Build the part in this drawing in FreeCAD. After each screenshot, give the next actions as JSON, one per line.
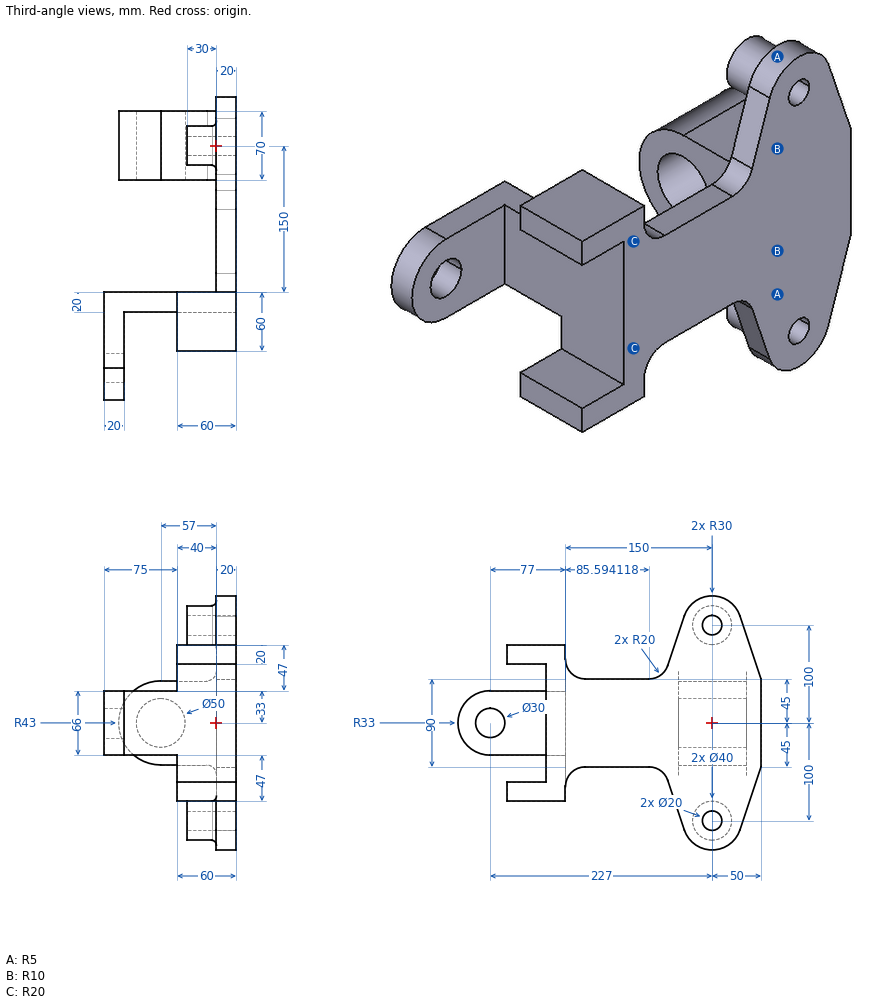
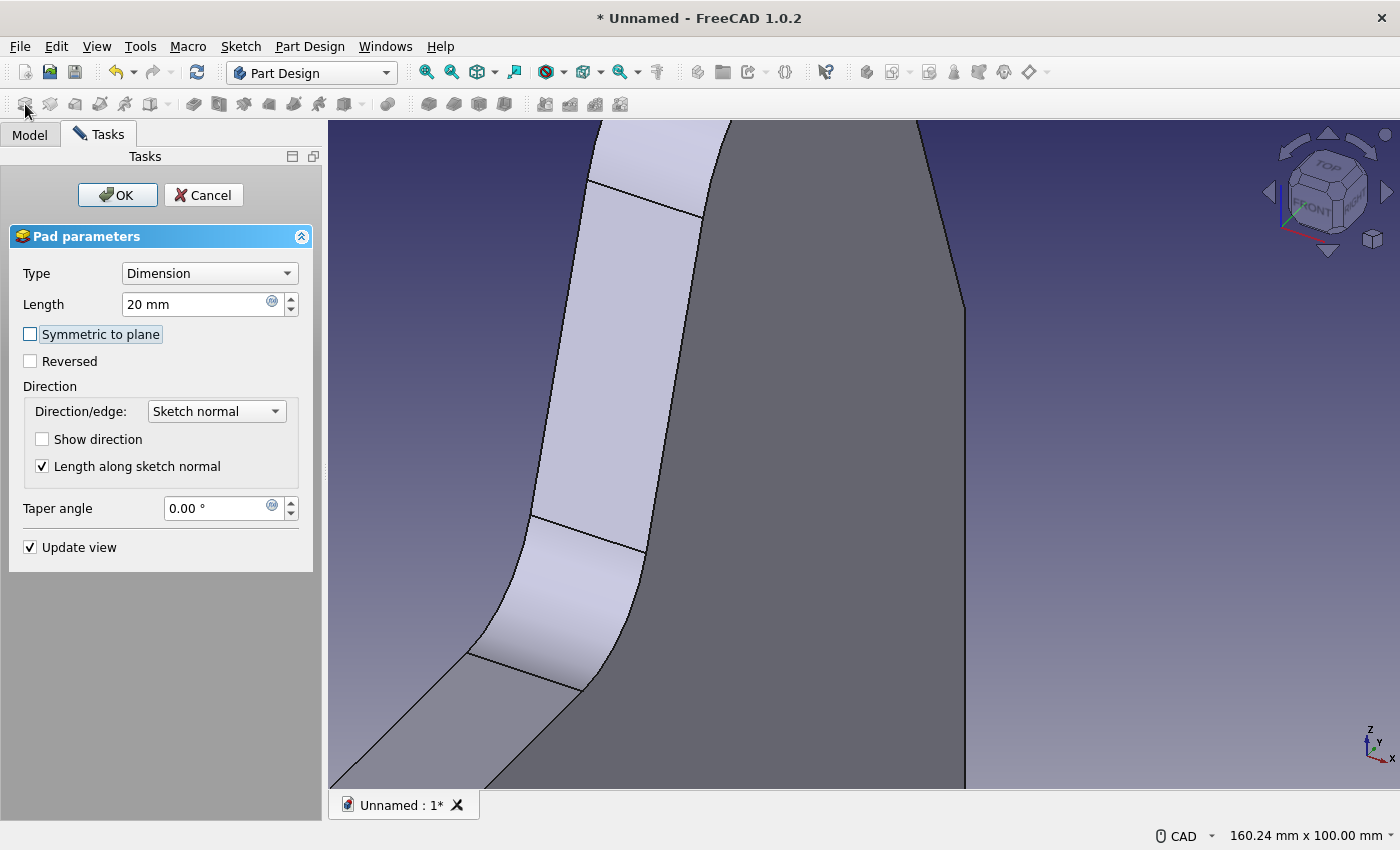
{"action": "left_click", "coordinate": [118, 195]}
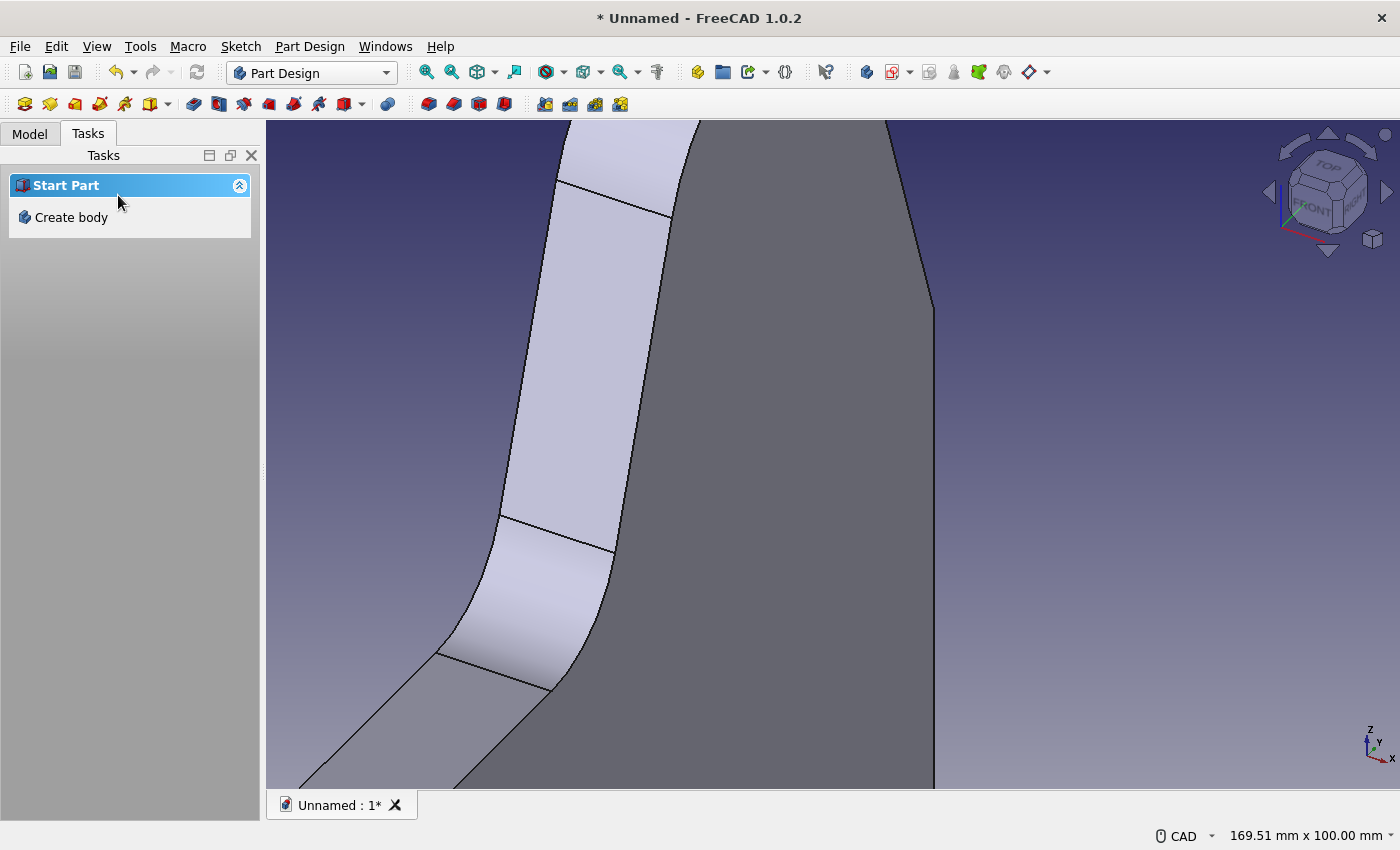
{"action": "left_click", "coordinate": [427, 72]}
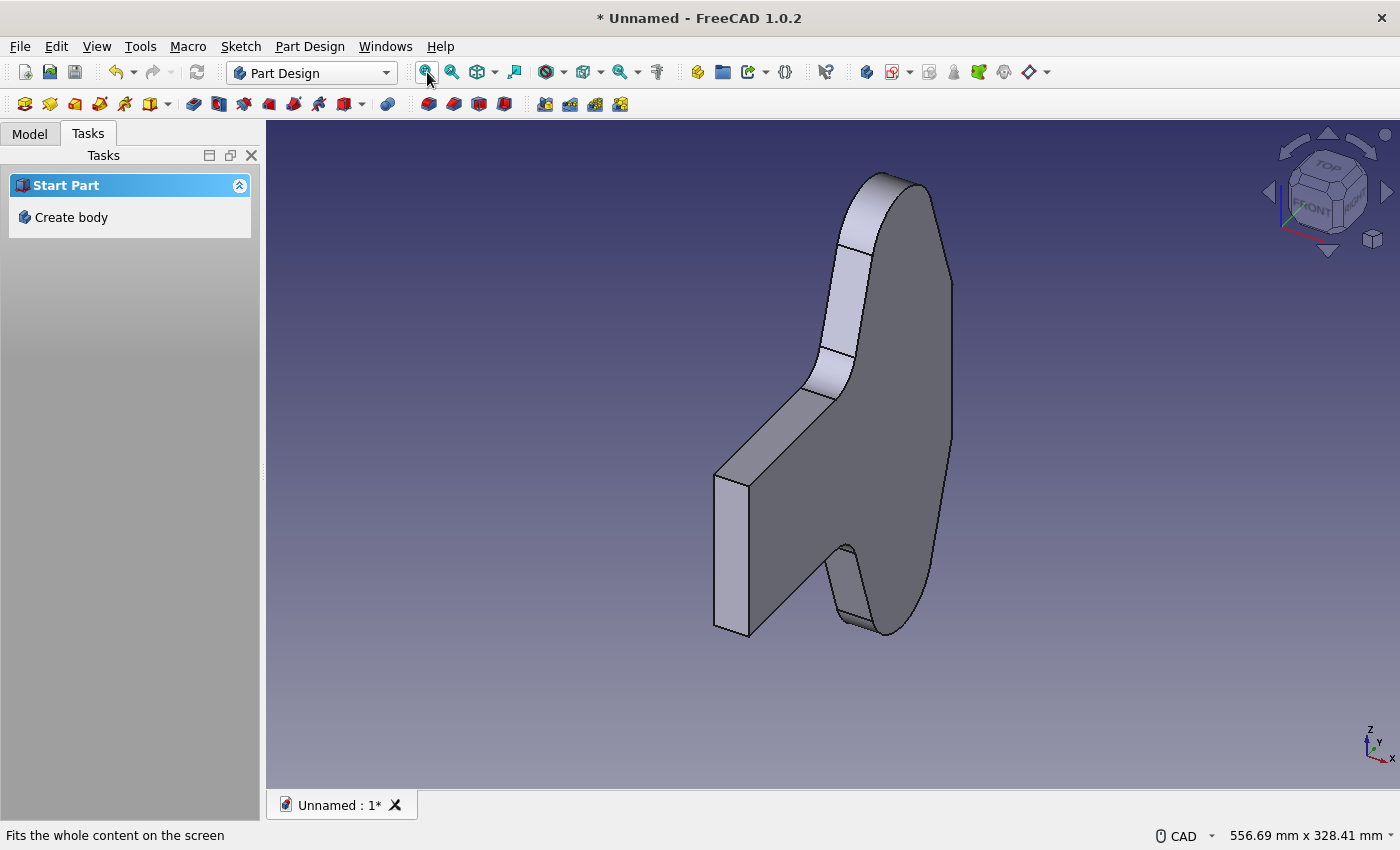
{"action": "left_click", "coordinate": [892, 72]}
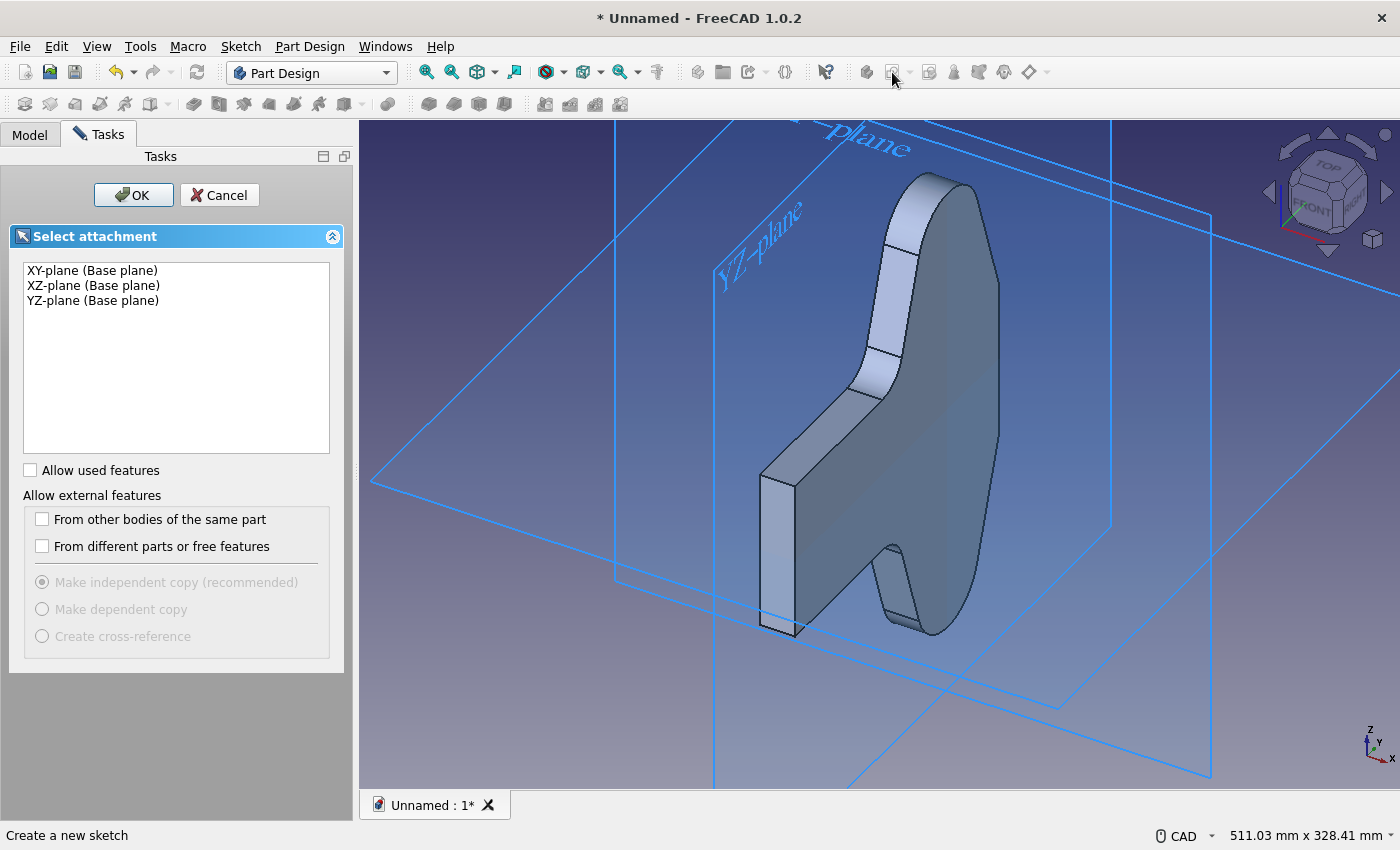
{"action": "left_click", "coordinate": [84, 300]}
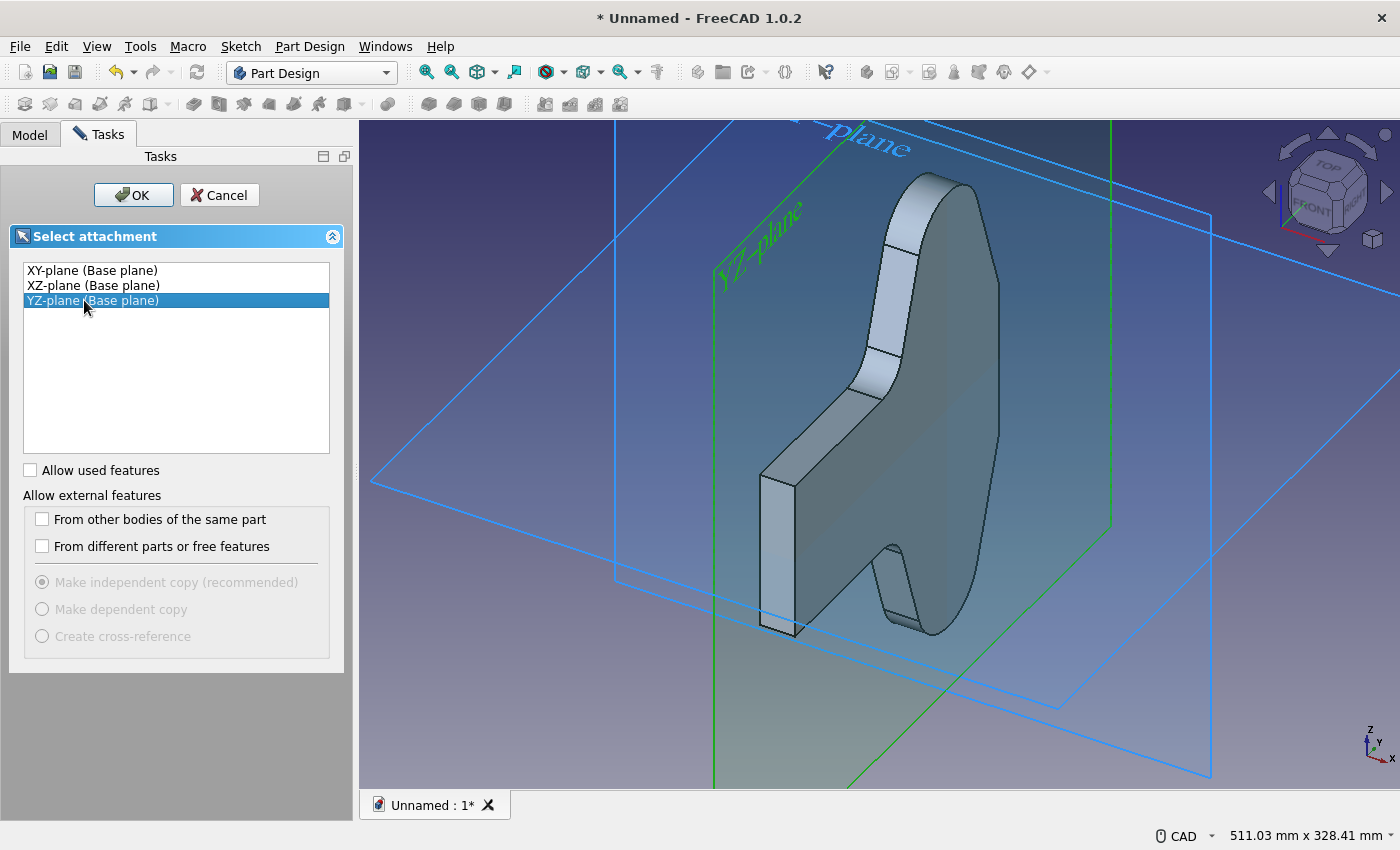
{"action": "left_click", "coordinate": [134, 195]}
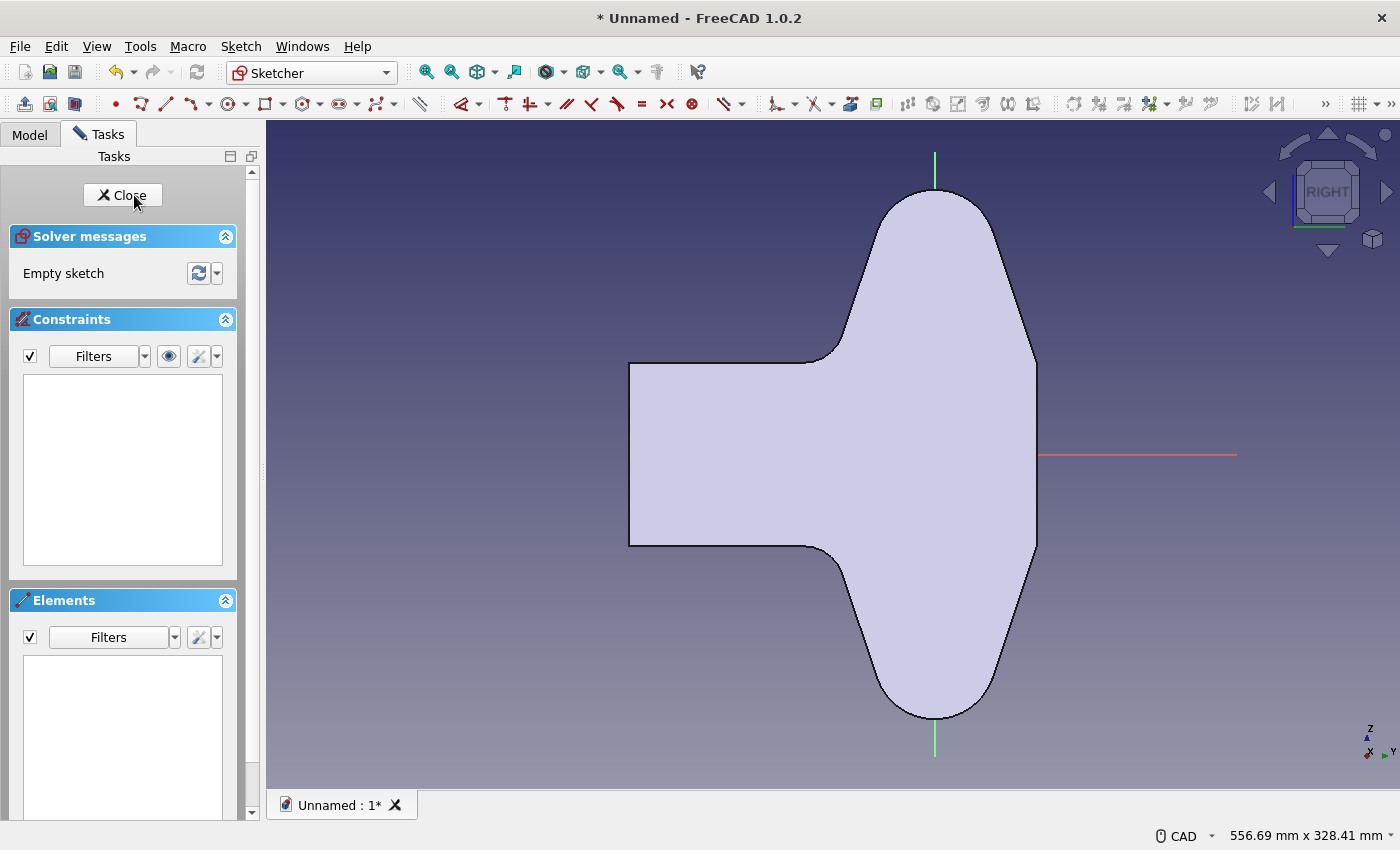
{"action": "key", "text": "q s"}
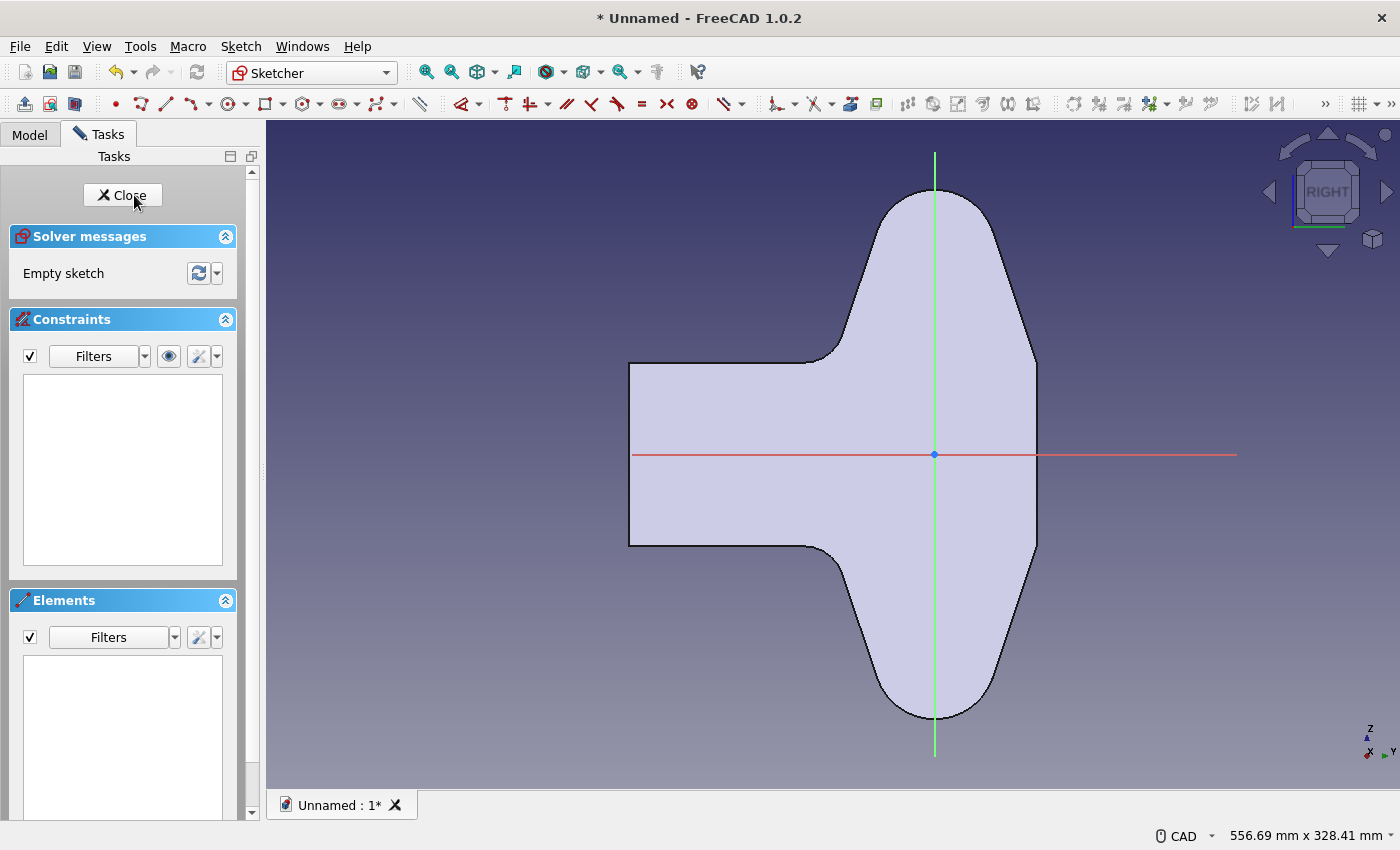
{"action": "left_click", "coordinate": [228, 104]}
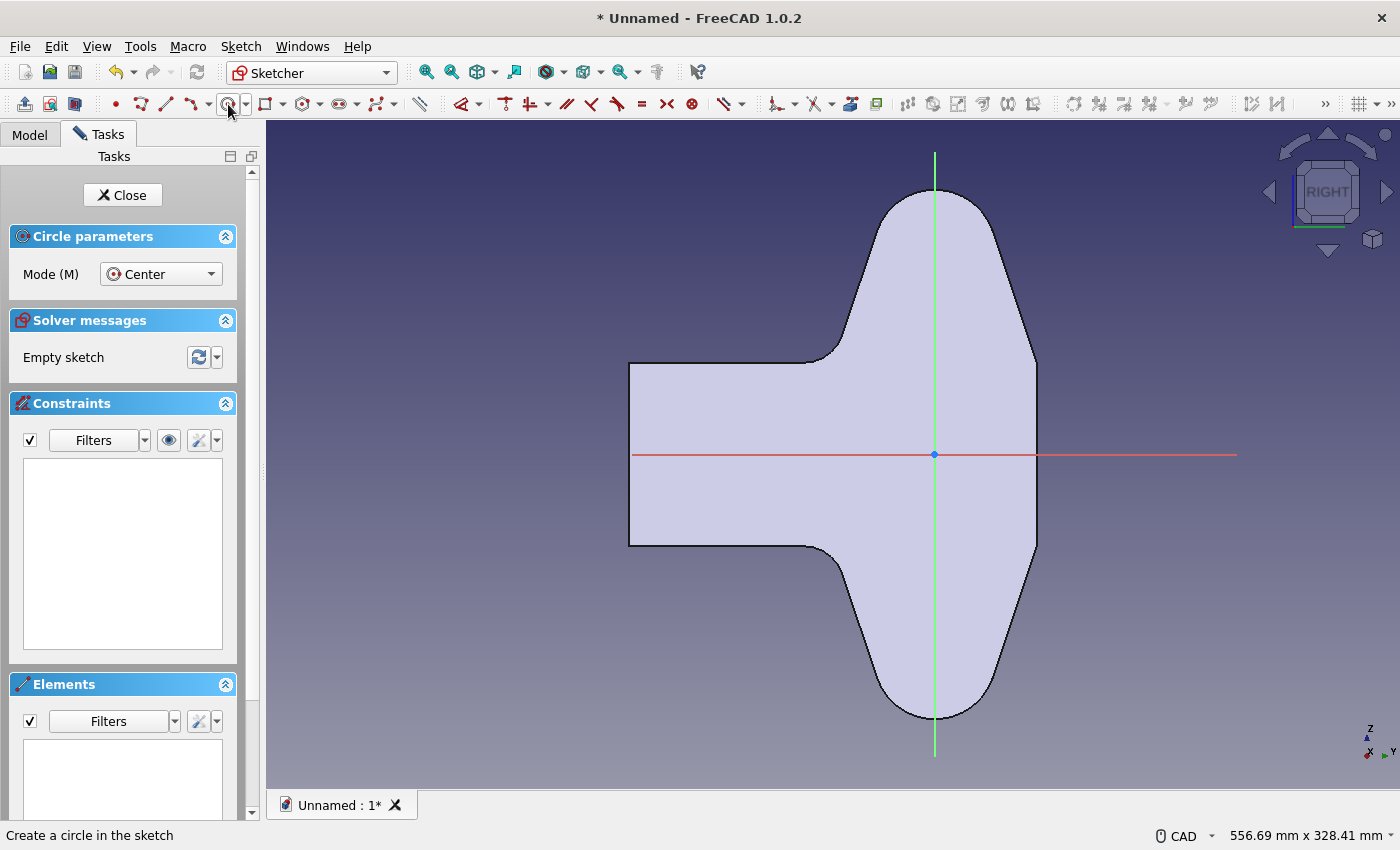
{"action": "left_click", "coordinate": [935, 658]}
{"action": "left_click", "coordinate": [964, 629]}